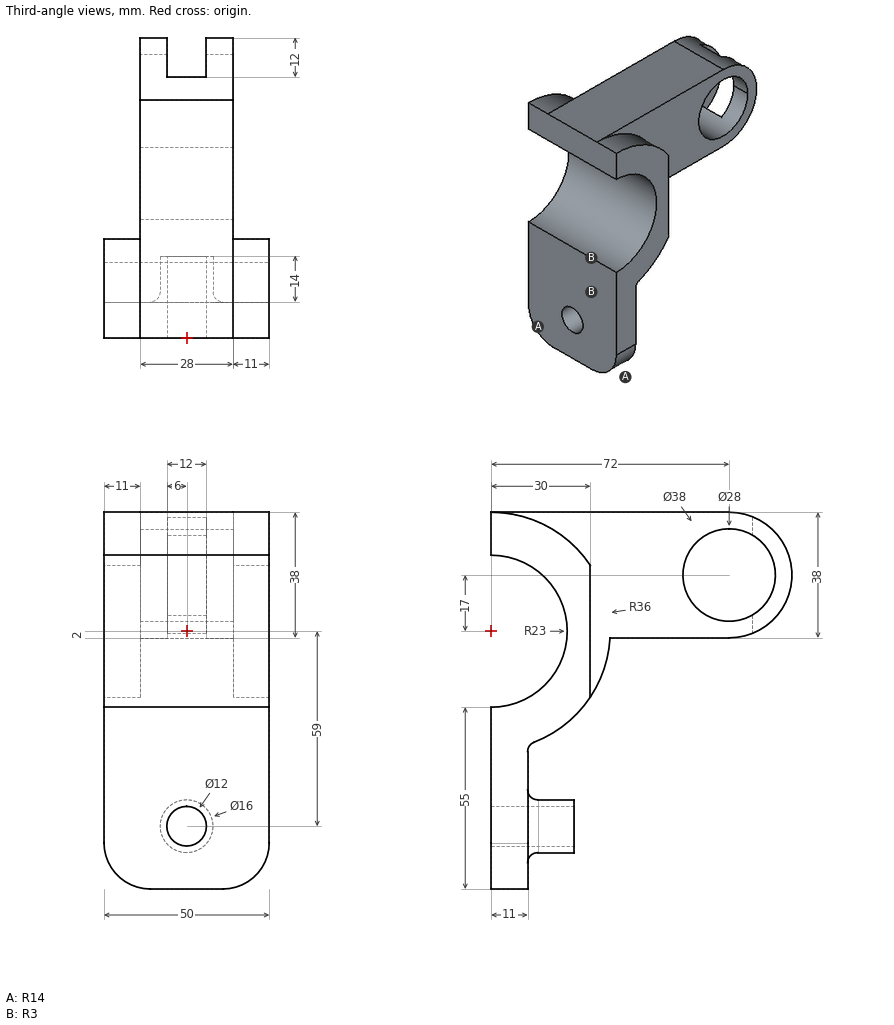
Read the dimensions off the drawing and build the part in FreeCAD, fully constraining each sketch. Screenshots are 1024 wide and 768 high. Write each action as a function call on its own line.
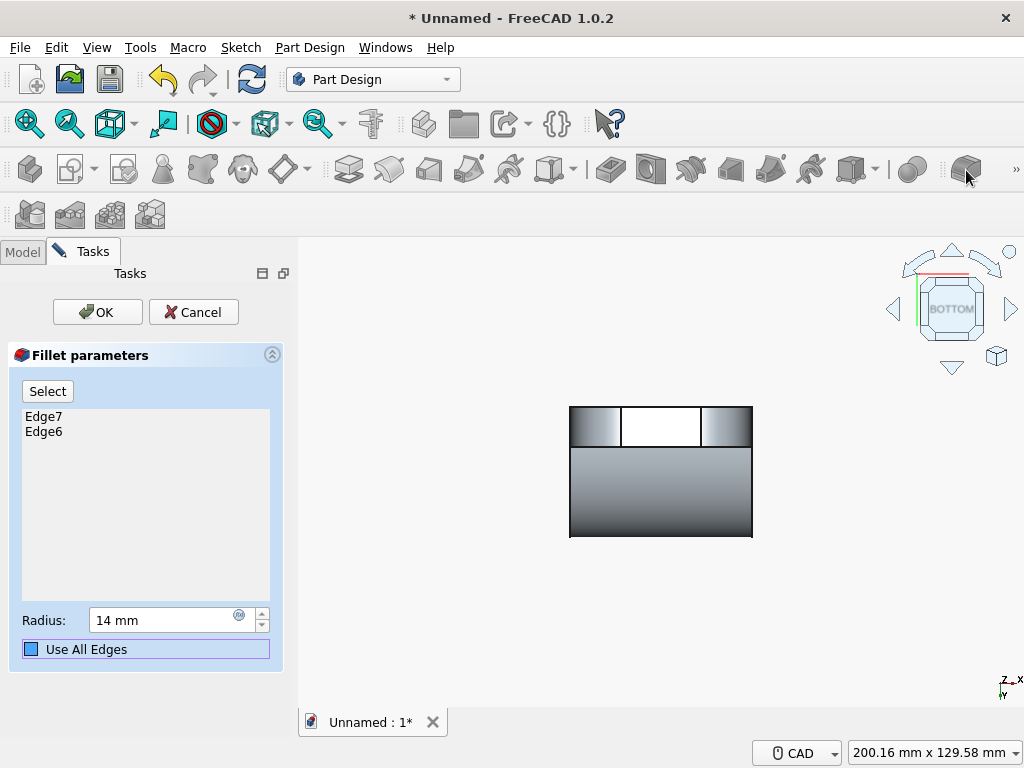
click(98, 312)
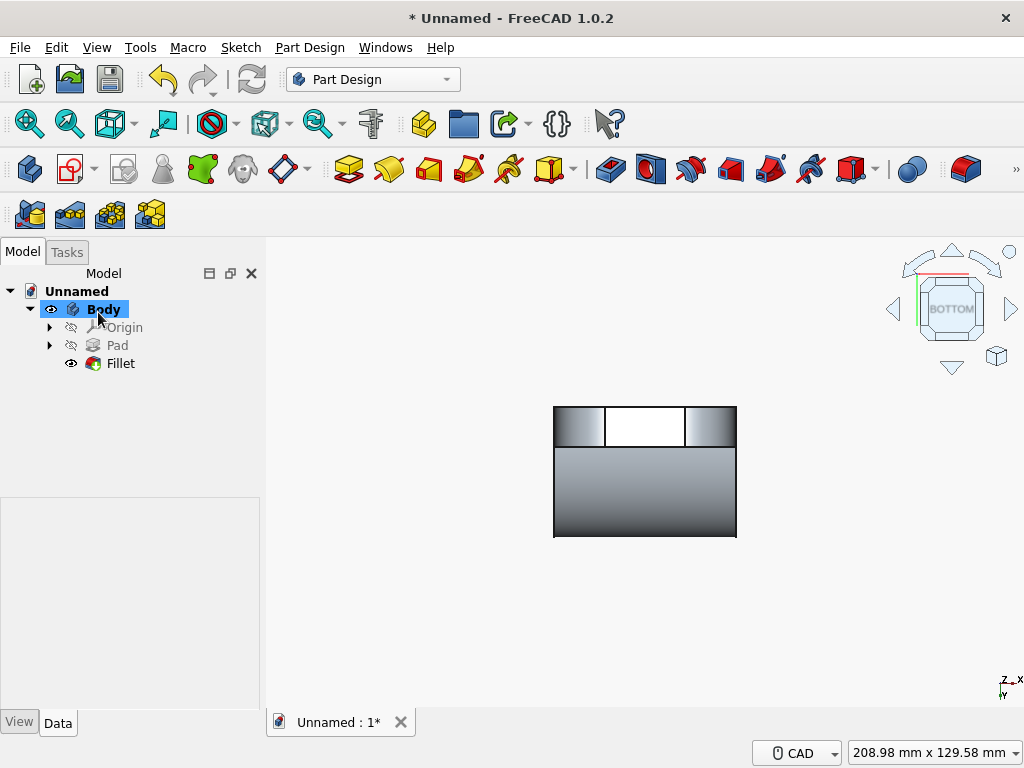
click(30, 124)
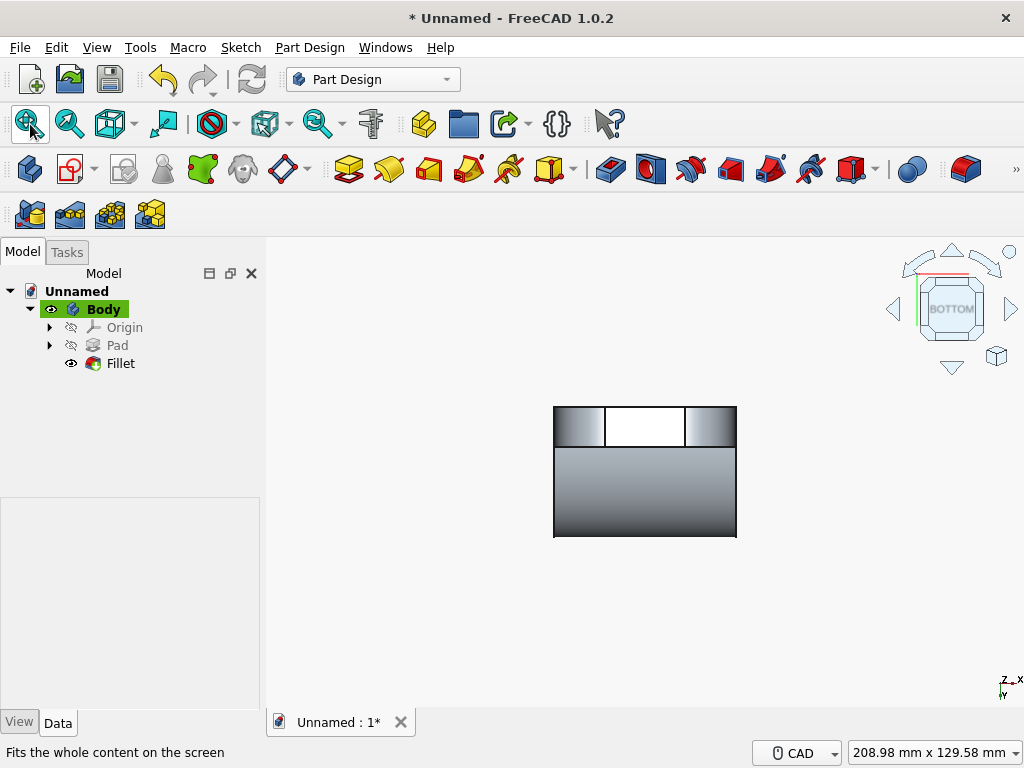
key(4)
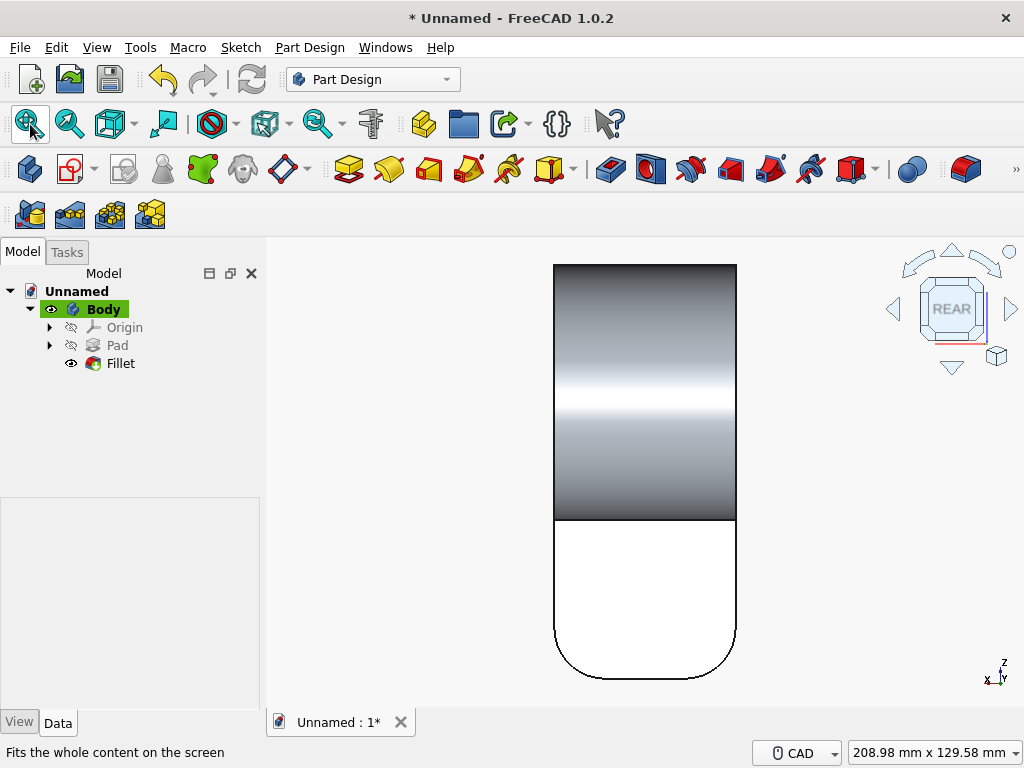
click(645, 598)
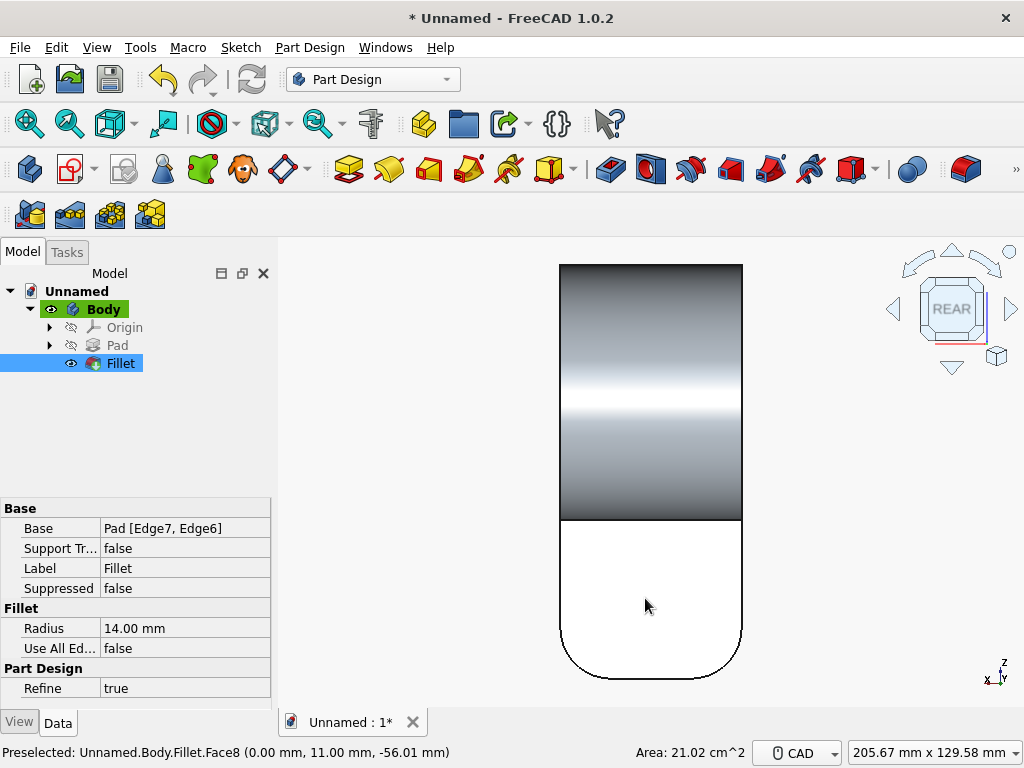
click(70, 170)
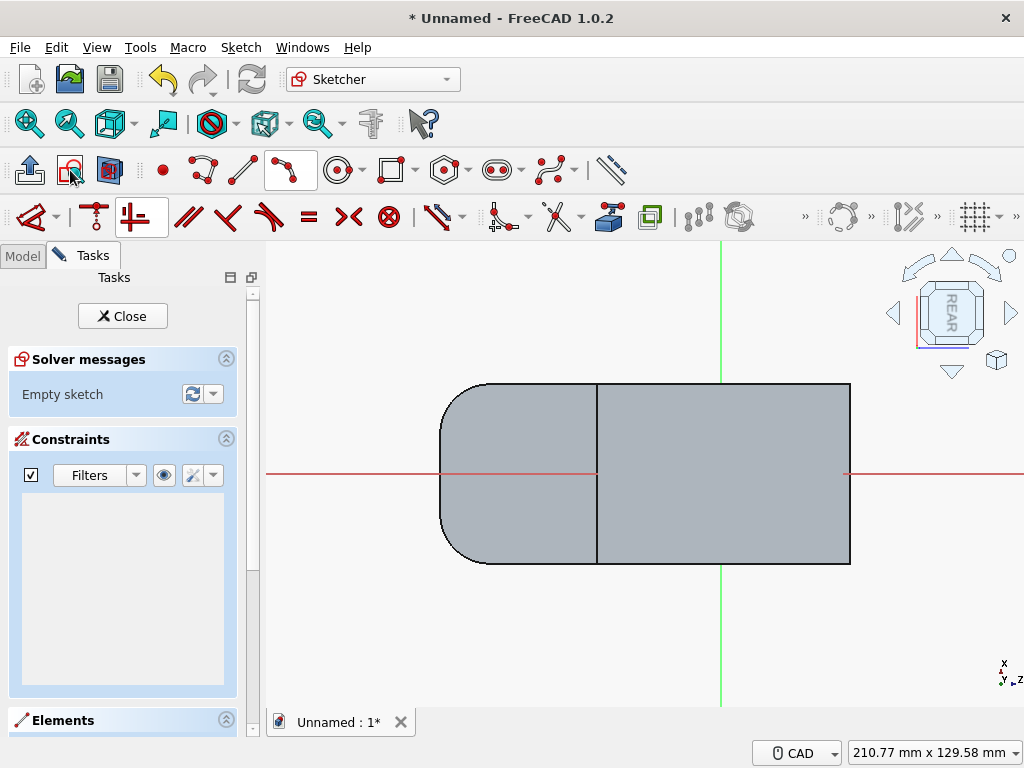
click(110, 170)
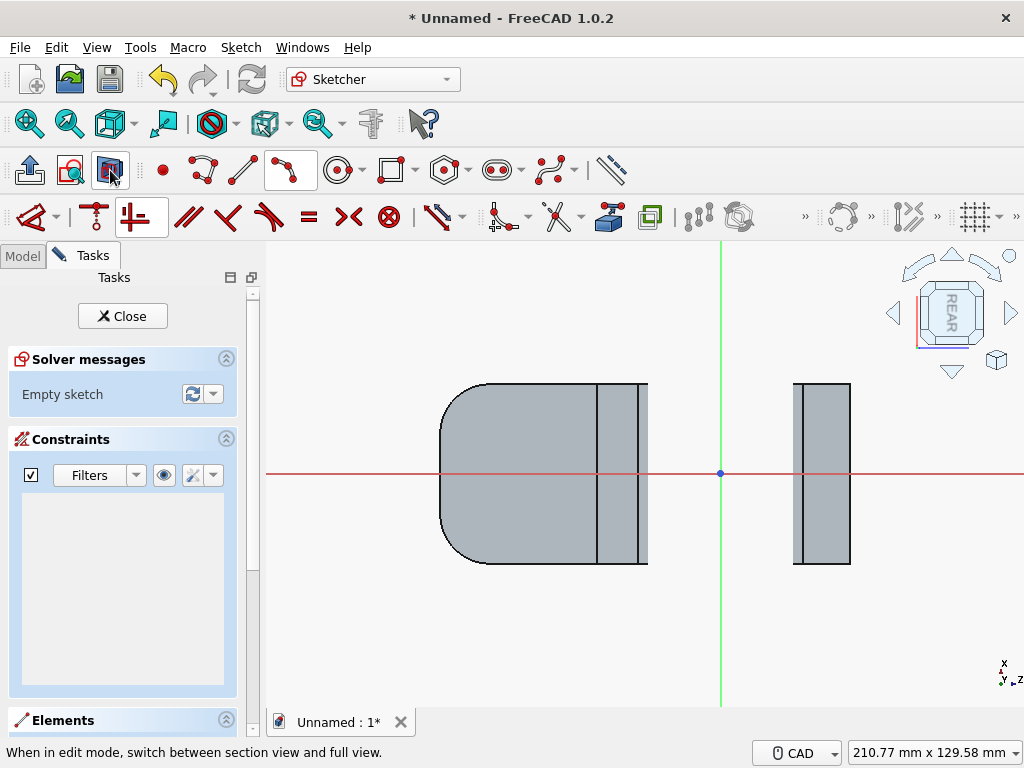
scroll(491, 474, up, 8)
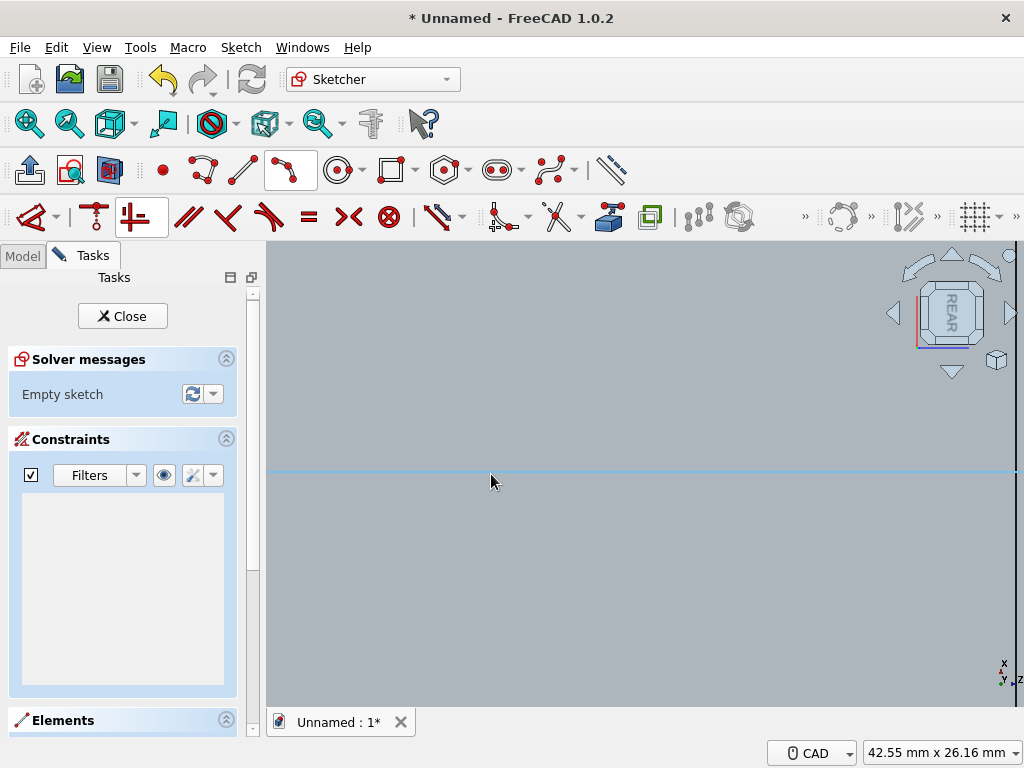
click(338, 170)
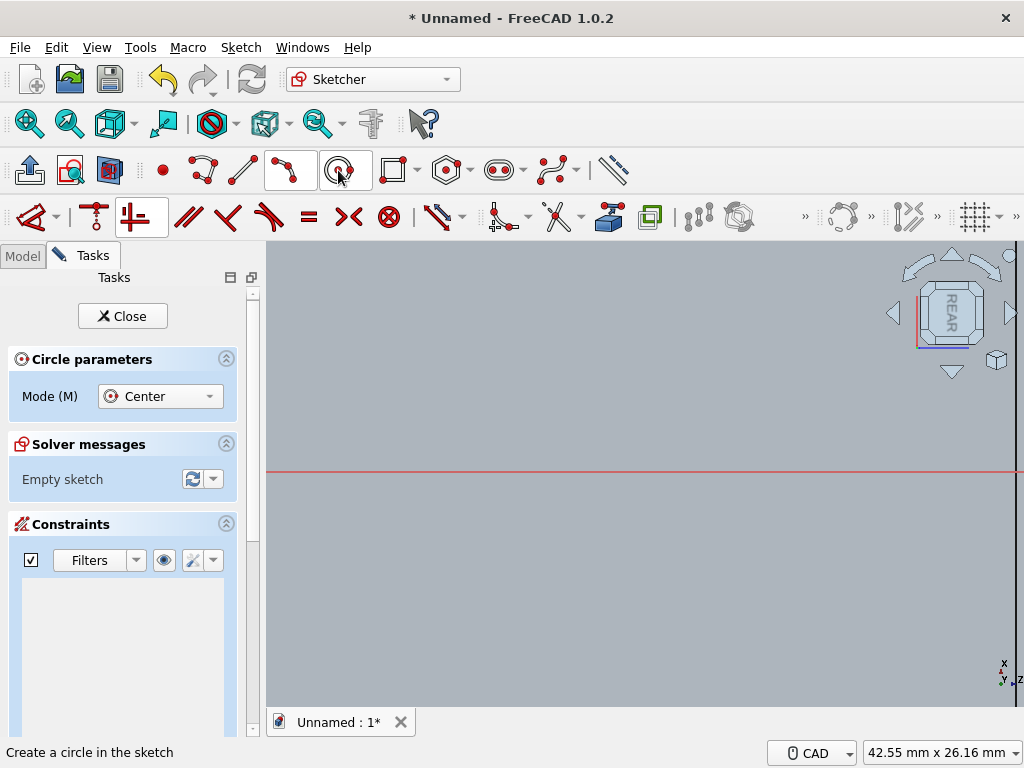
click(576, 472)
move(676, 371)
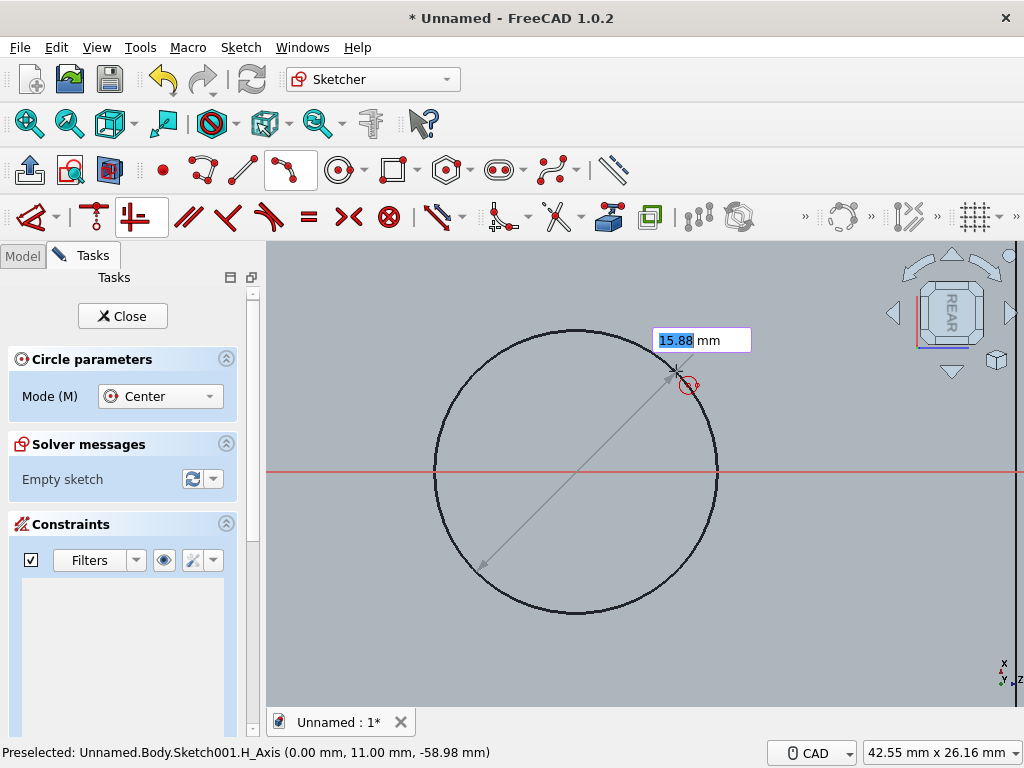
text(16)
key(Return)
key(Escape)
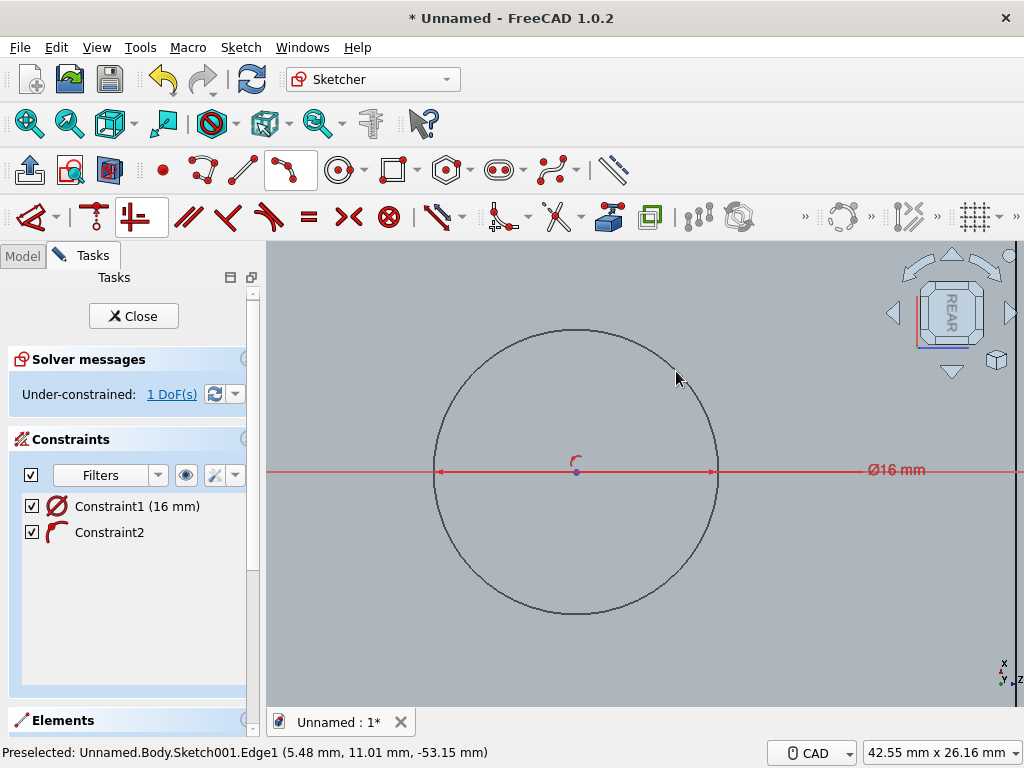
click(32, 218)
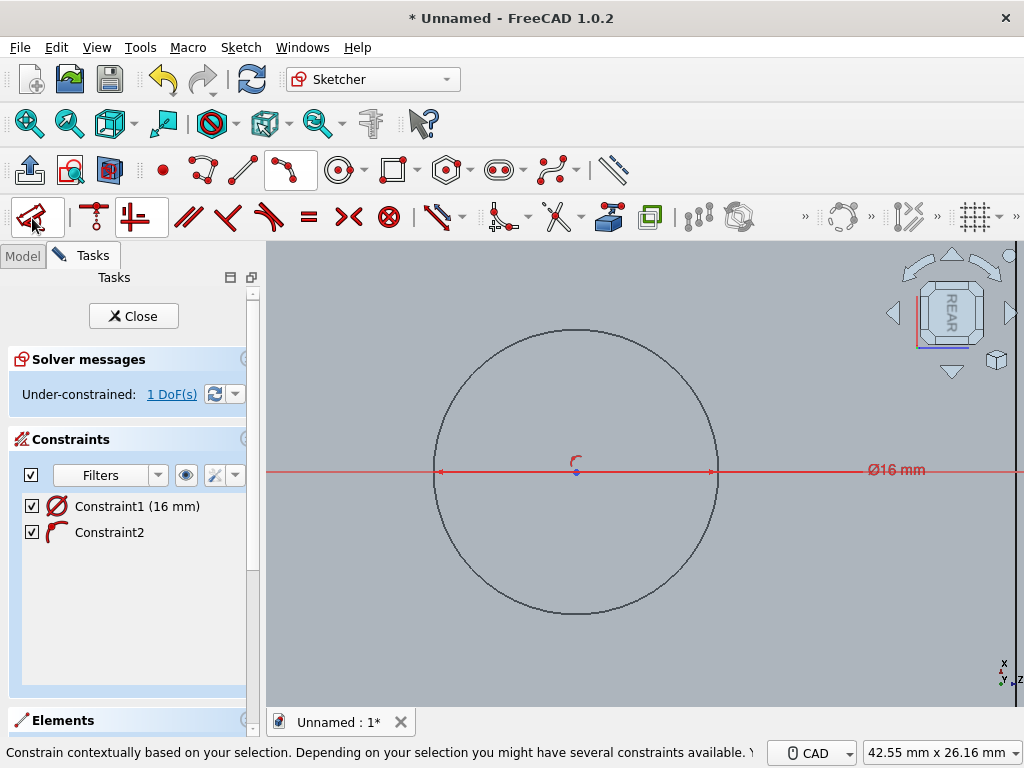
click(576, 472)
click(652, 506)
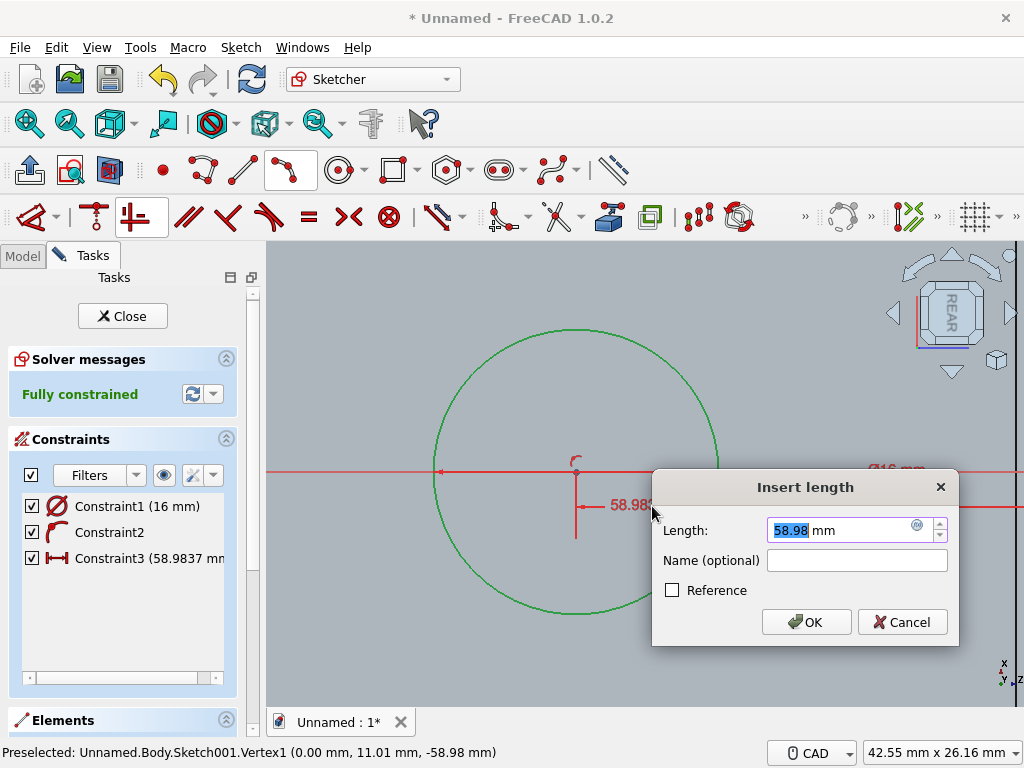
text(59)
key(Return)
key(Escape)